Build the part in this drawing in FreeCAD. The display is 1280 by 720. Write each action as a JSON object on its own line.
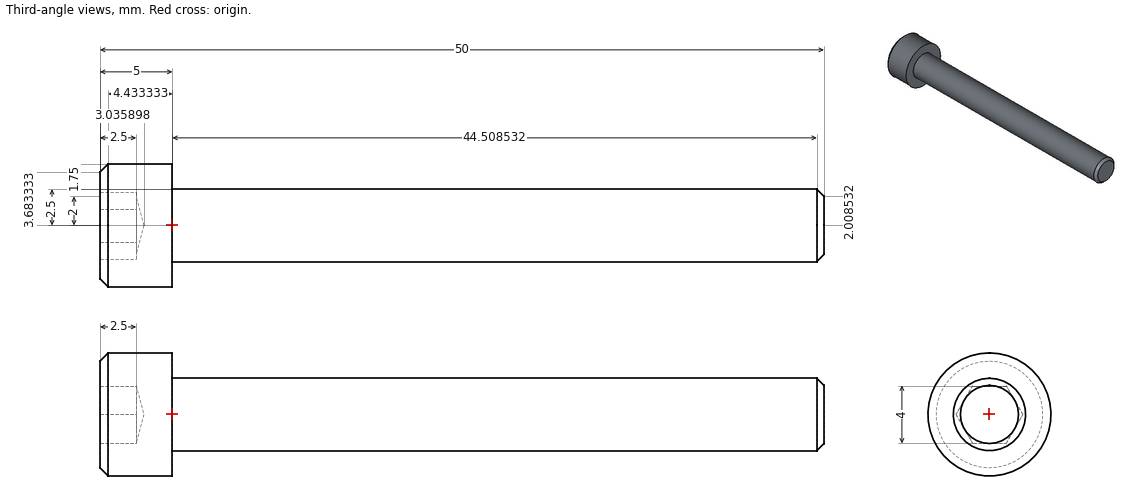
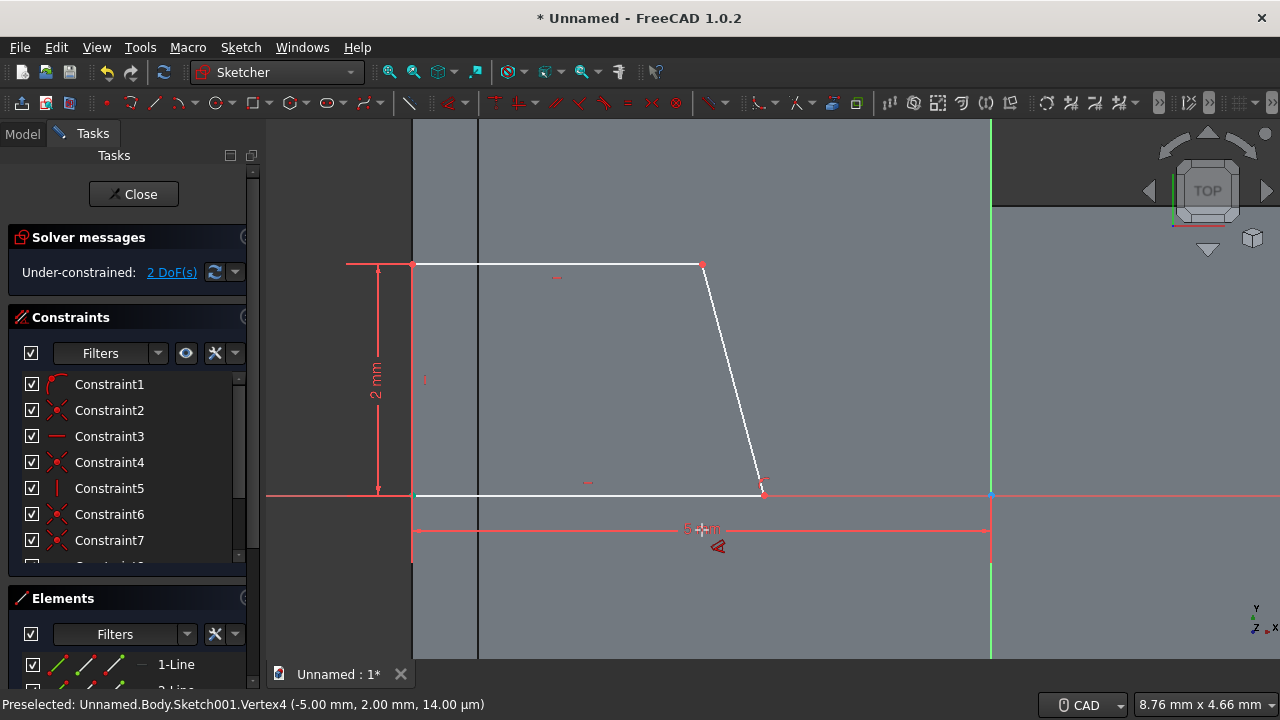
{"action": "left_click", "coordinate": [615, 264]}
{"action": "left_click", "coordinate": [557, 230]}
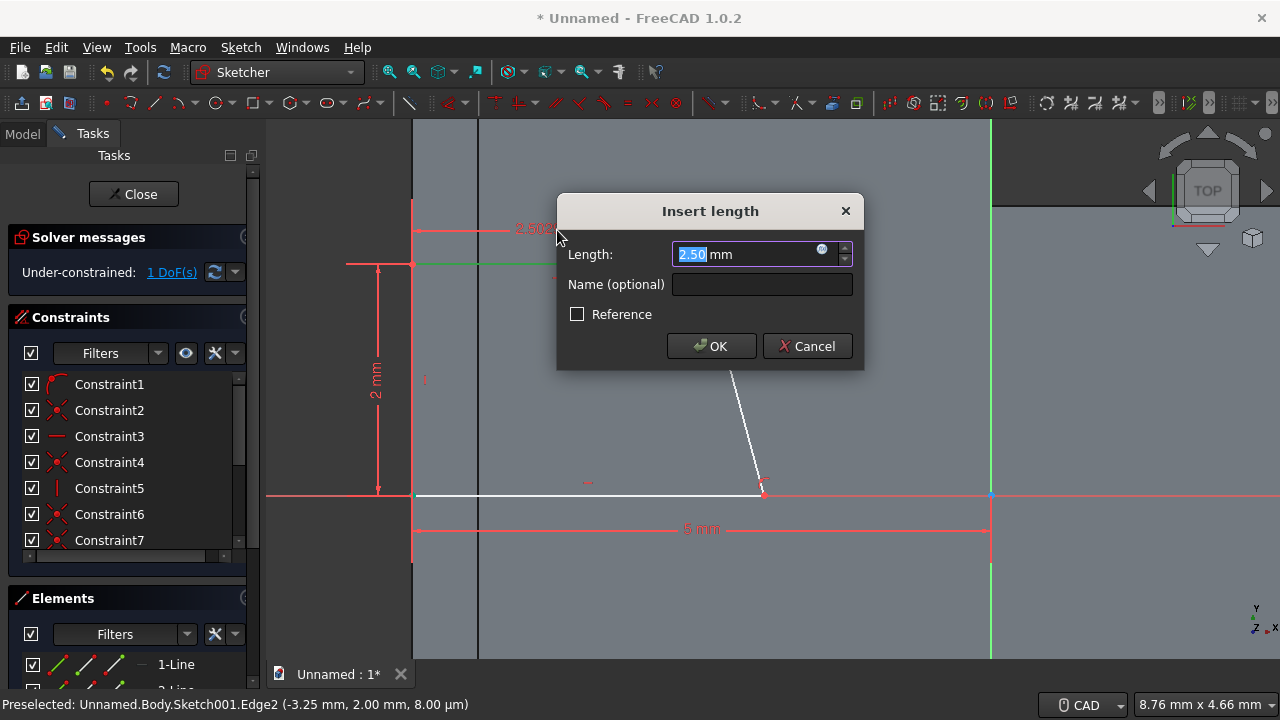
{"action": "type", "text": "2.5"}
{"action": "key", "text": "Return"}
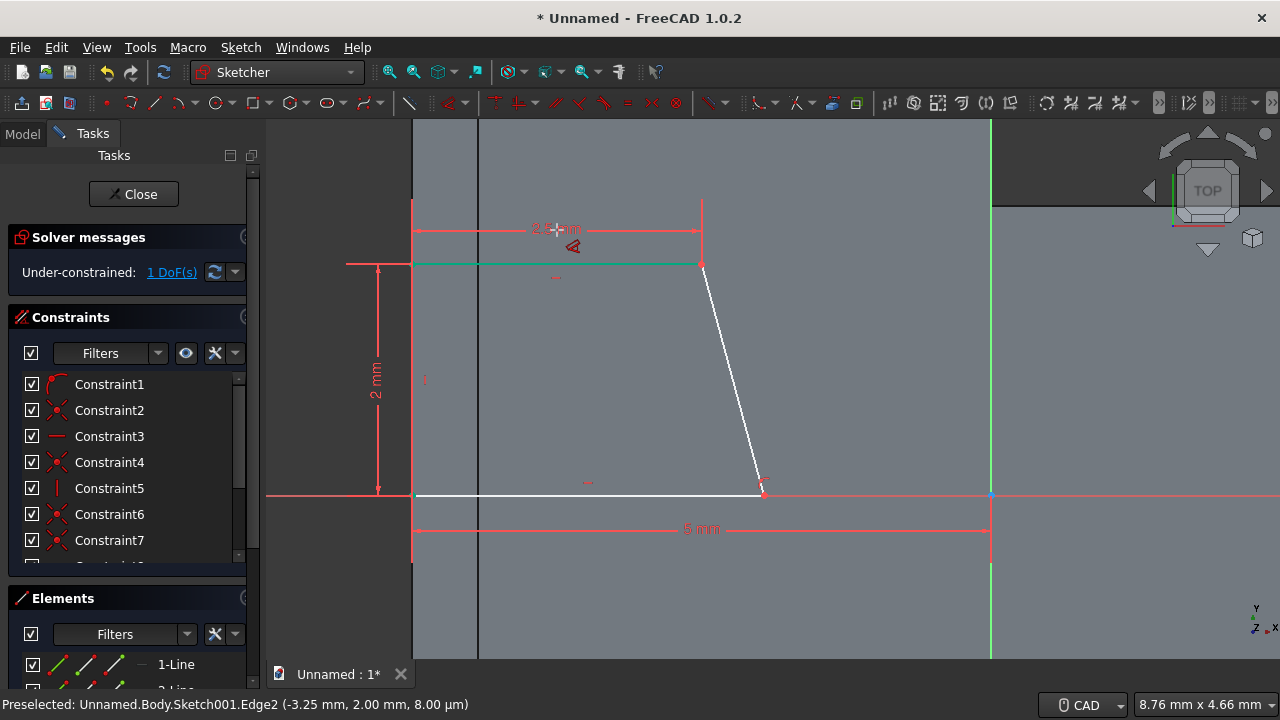
{"action": "left_click", "coordinate": [518, 496]}
{"action": "left_click", "coordinate": [588, 530]}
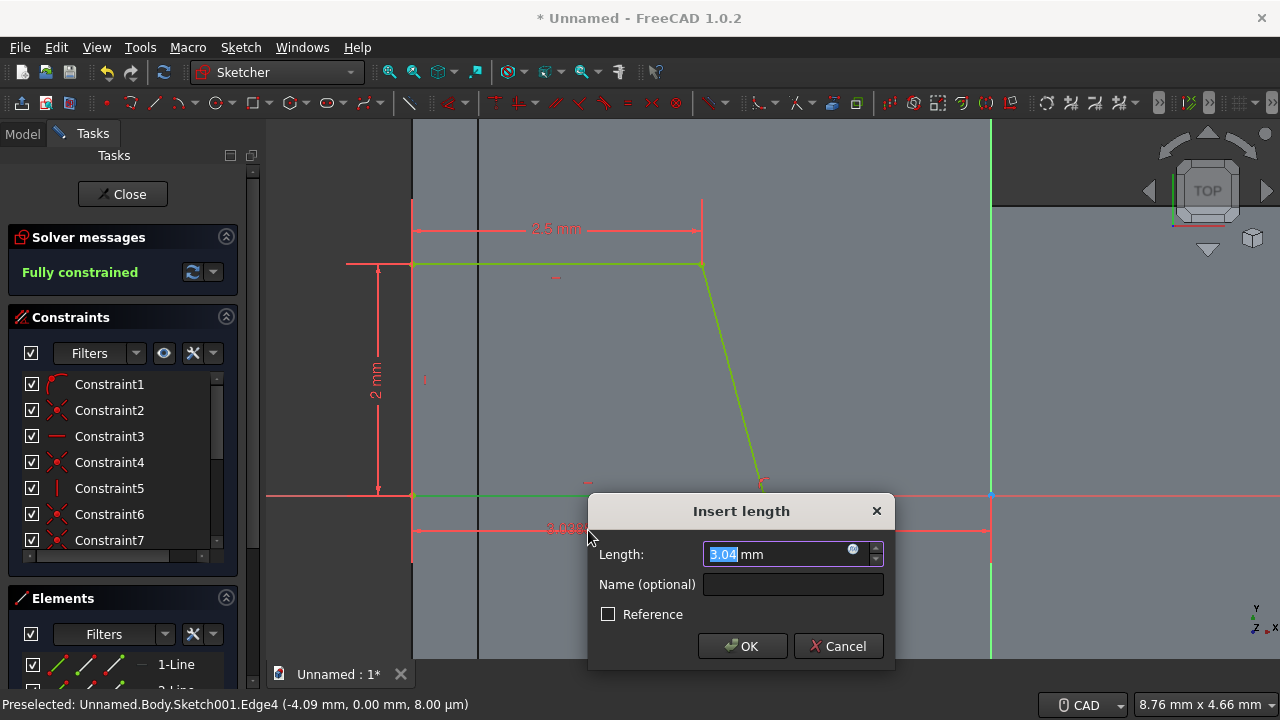
{"action": "type", "text": "3.035898"}
{"action": "key", "text": "Return"}
{"action": "key", "text": "Escape"}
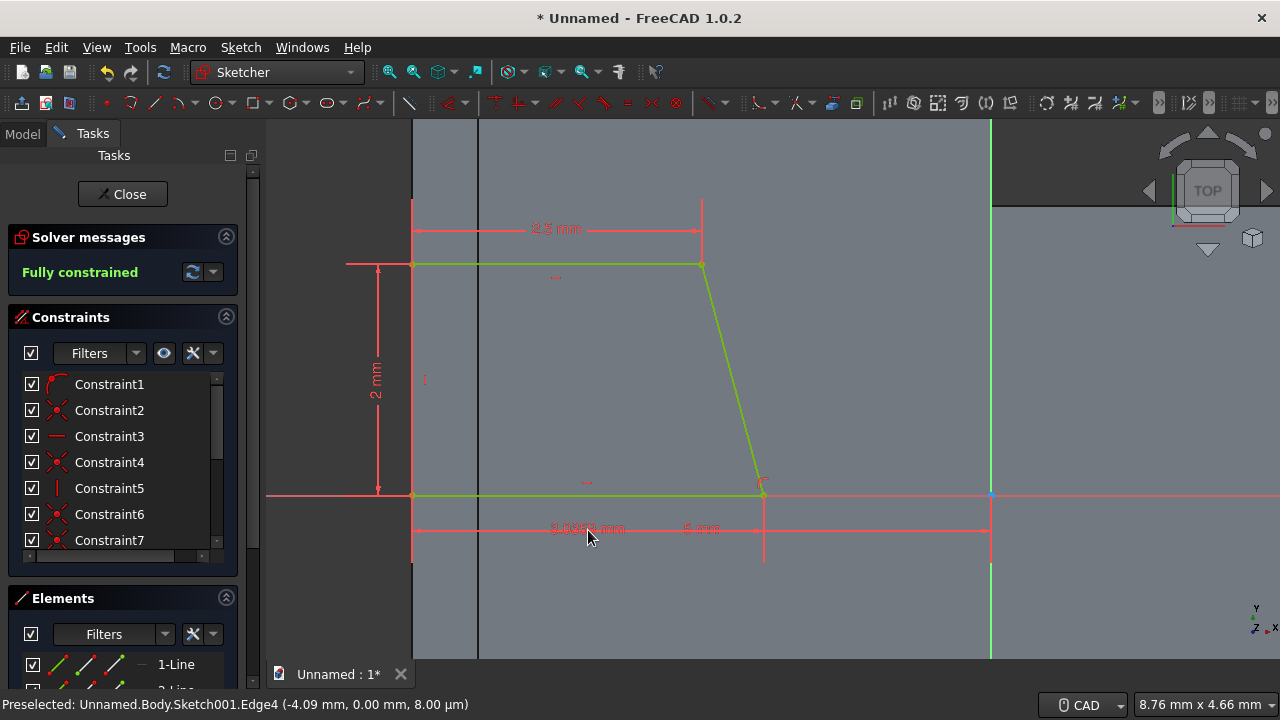
{"action": "left_click", "coordinate": [123, 194]}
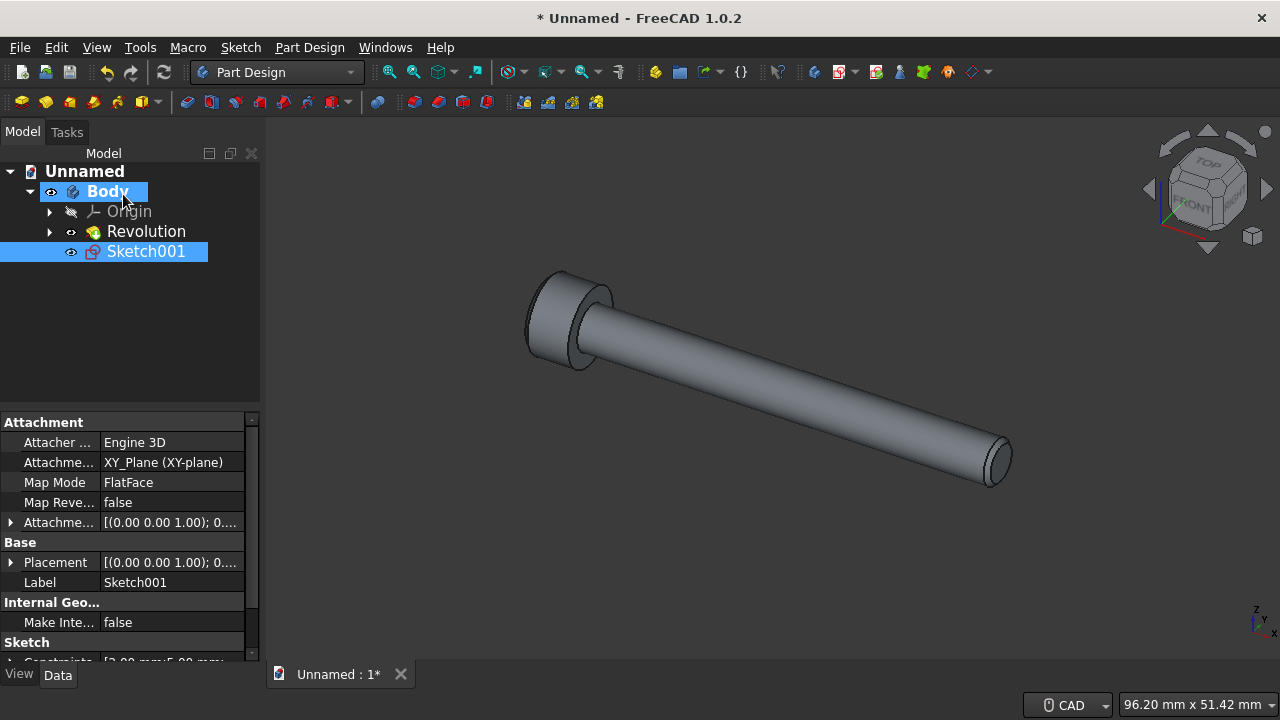
{"action": "left_click", "coordinate": [236, 102]}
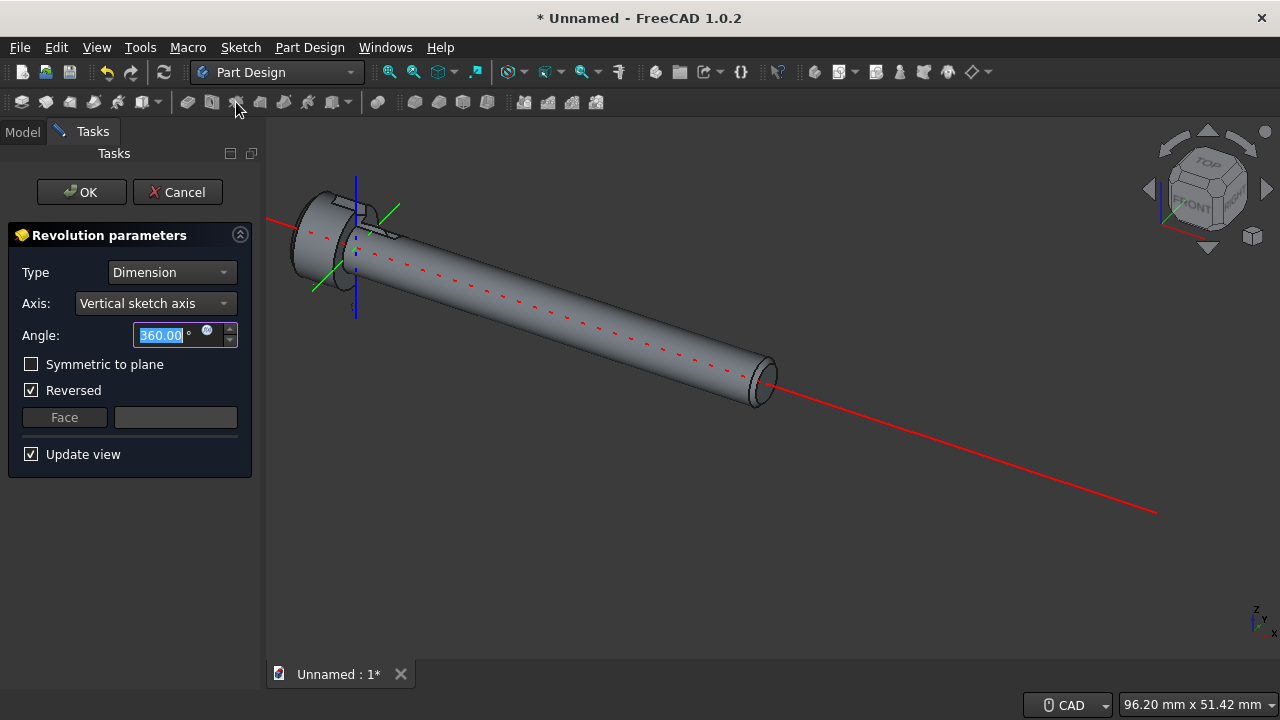
{"action": "left_click", "coordinate": [156, 304]}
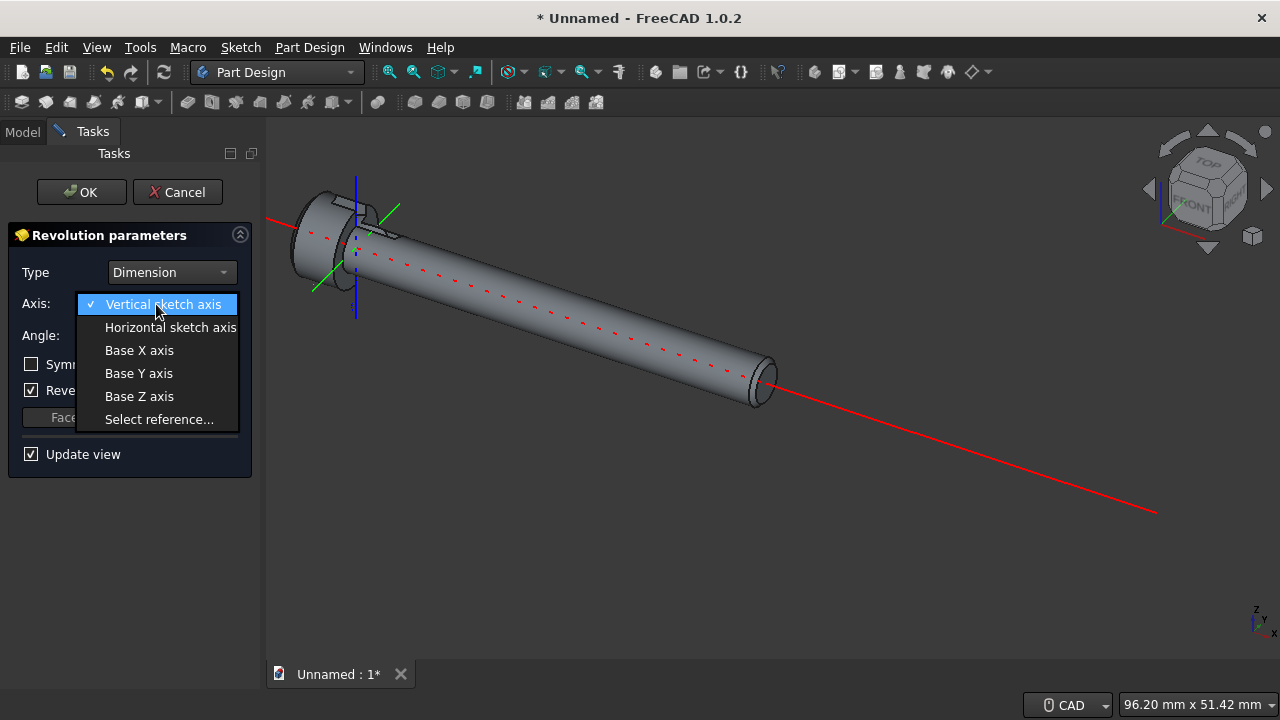
{"action": "left_click", "coordinate": [156, 328]}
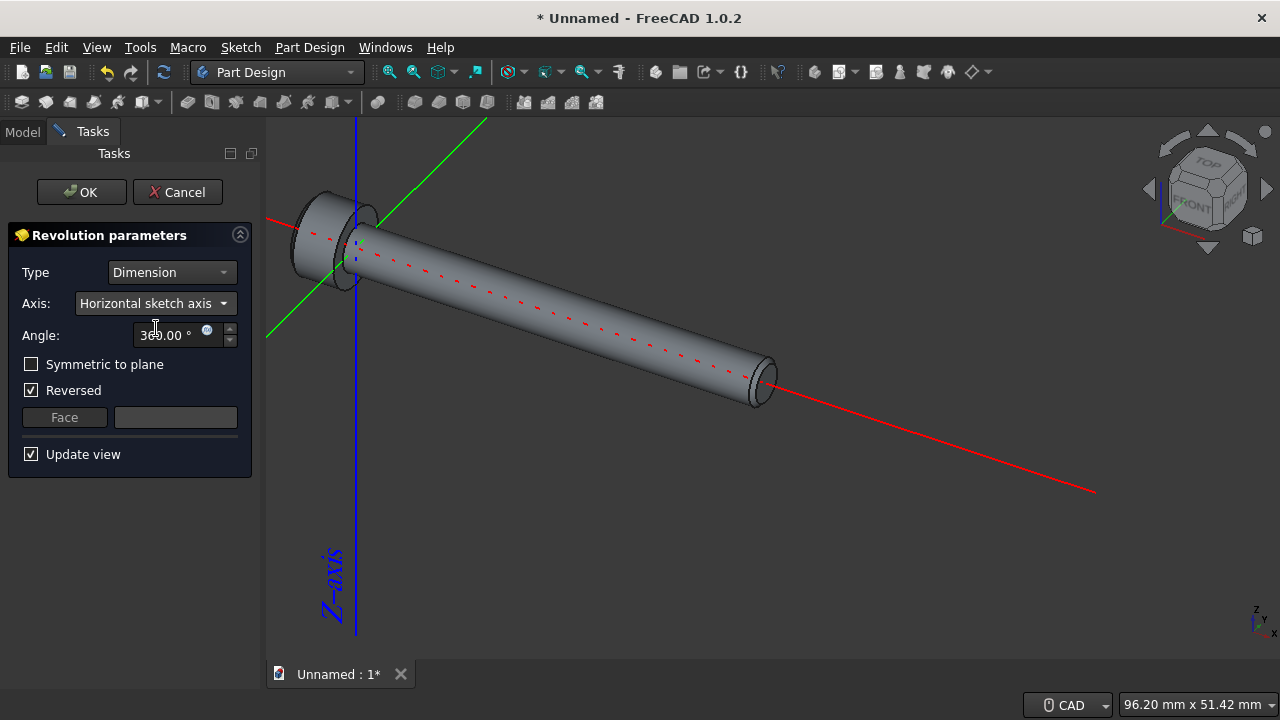
{"action": "left_click", "coordinate": [82, 192]}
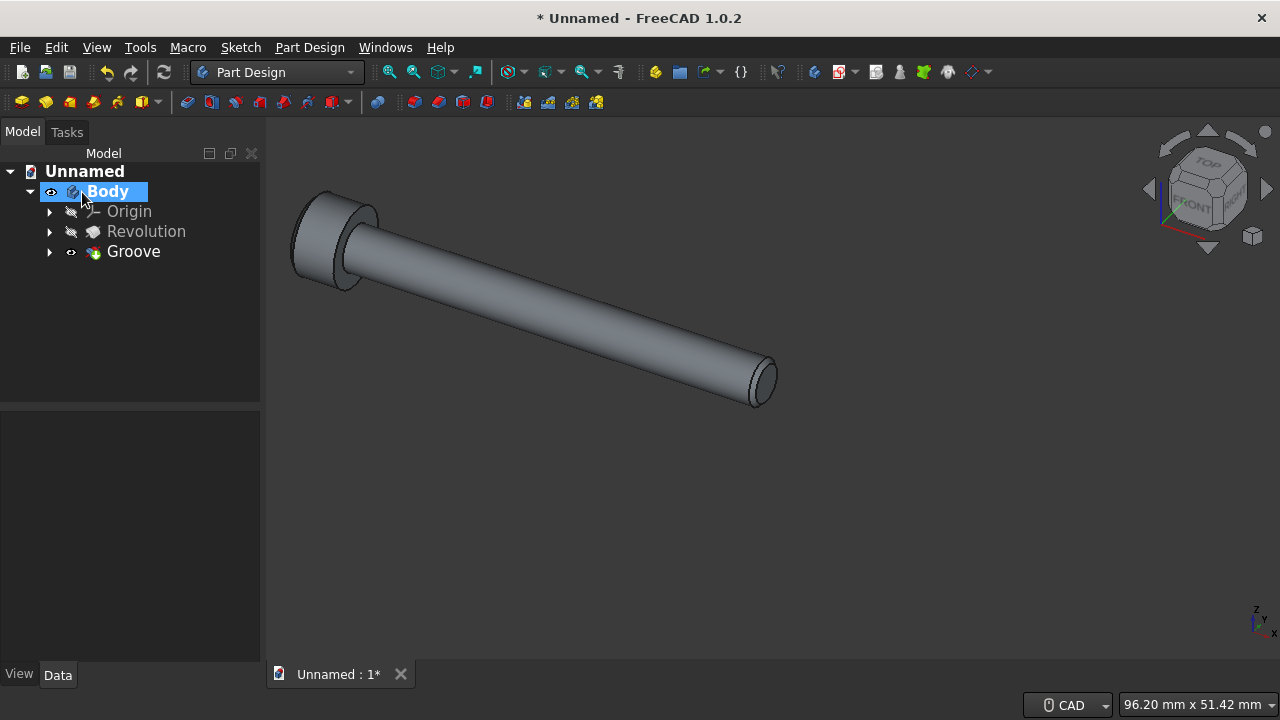
{"action": "key", "text": "6"}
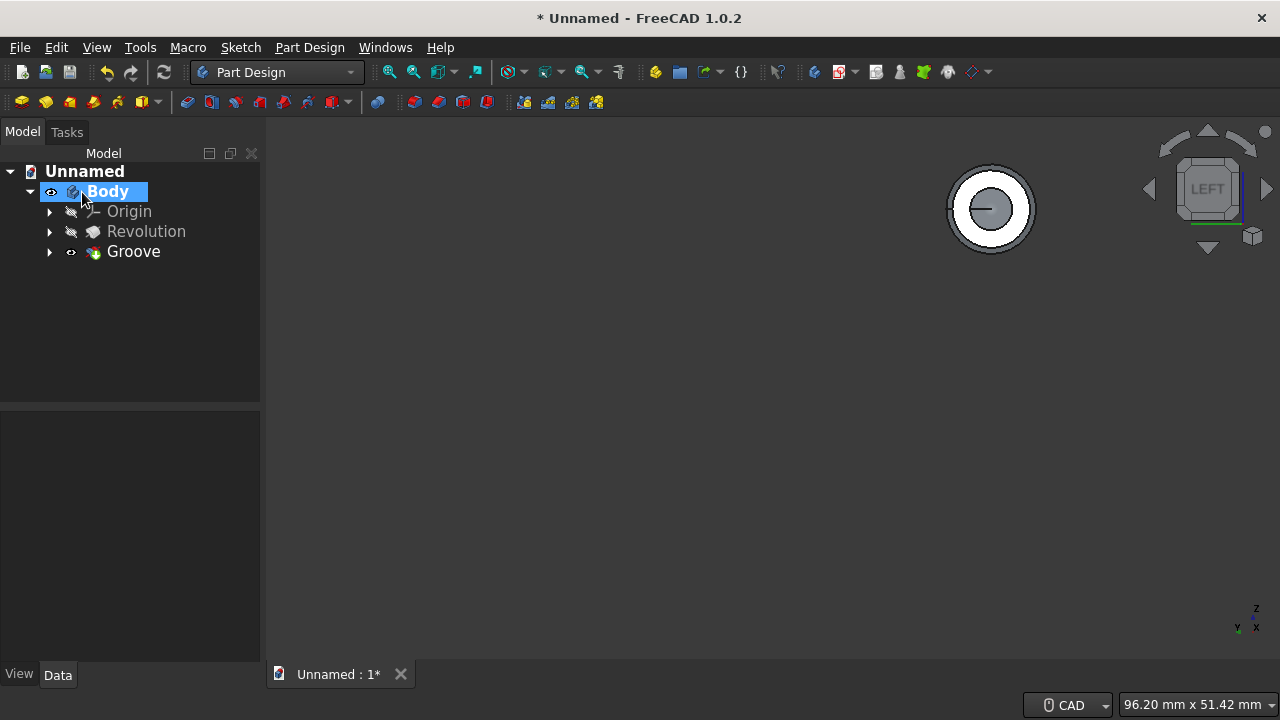
{"action": "left_click", "coordinate": [390, 72]}